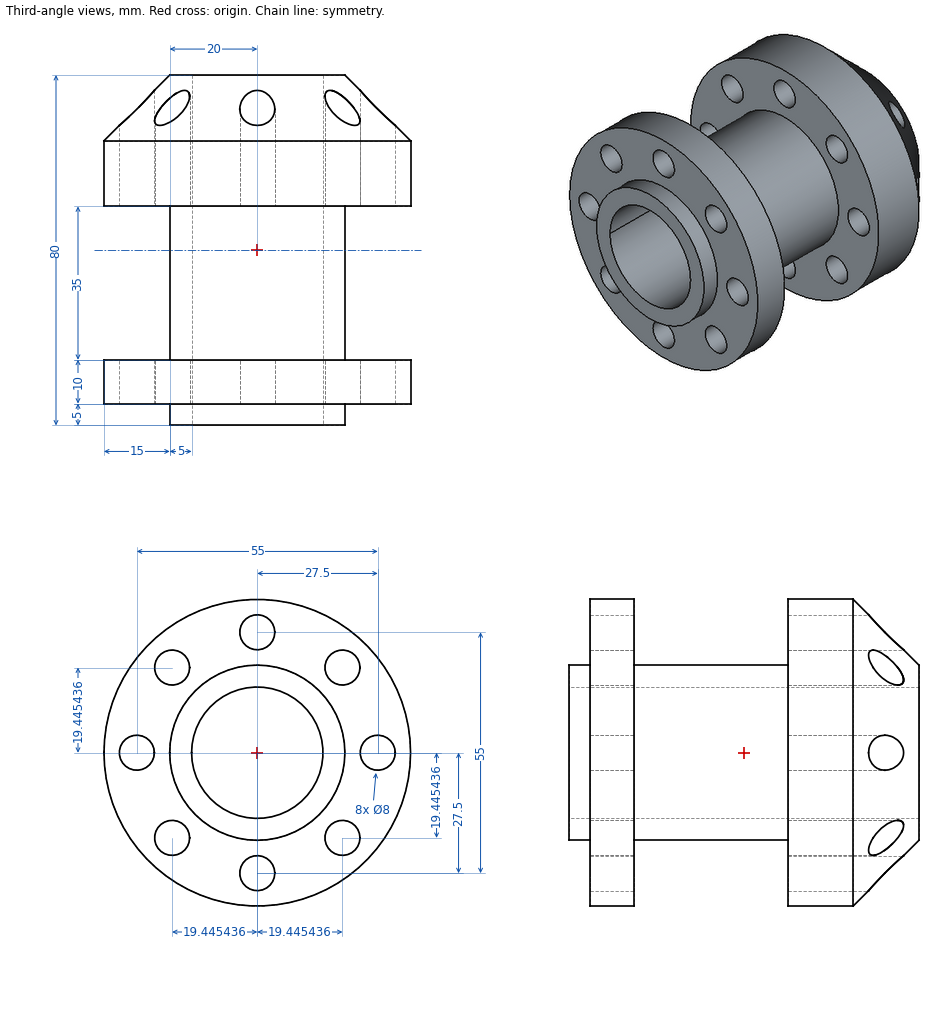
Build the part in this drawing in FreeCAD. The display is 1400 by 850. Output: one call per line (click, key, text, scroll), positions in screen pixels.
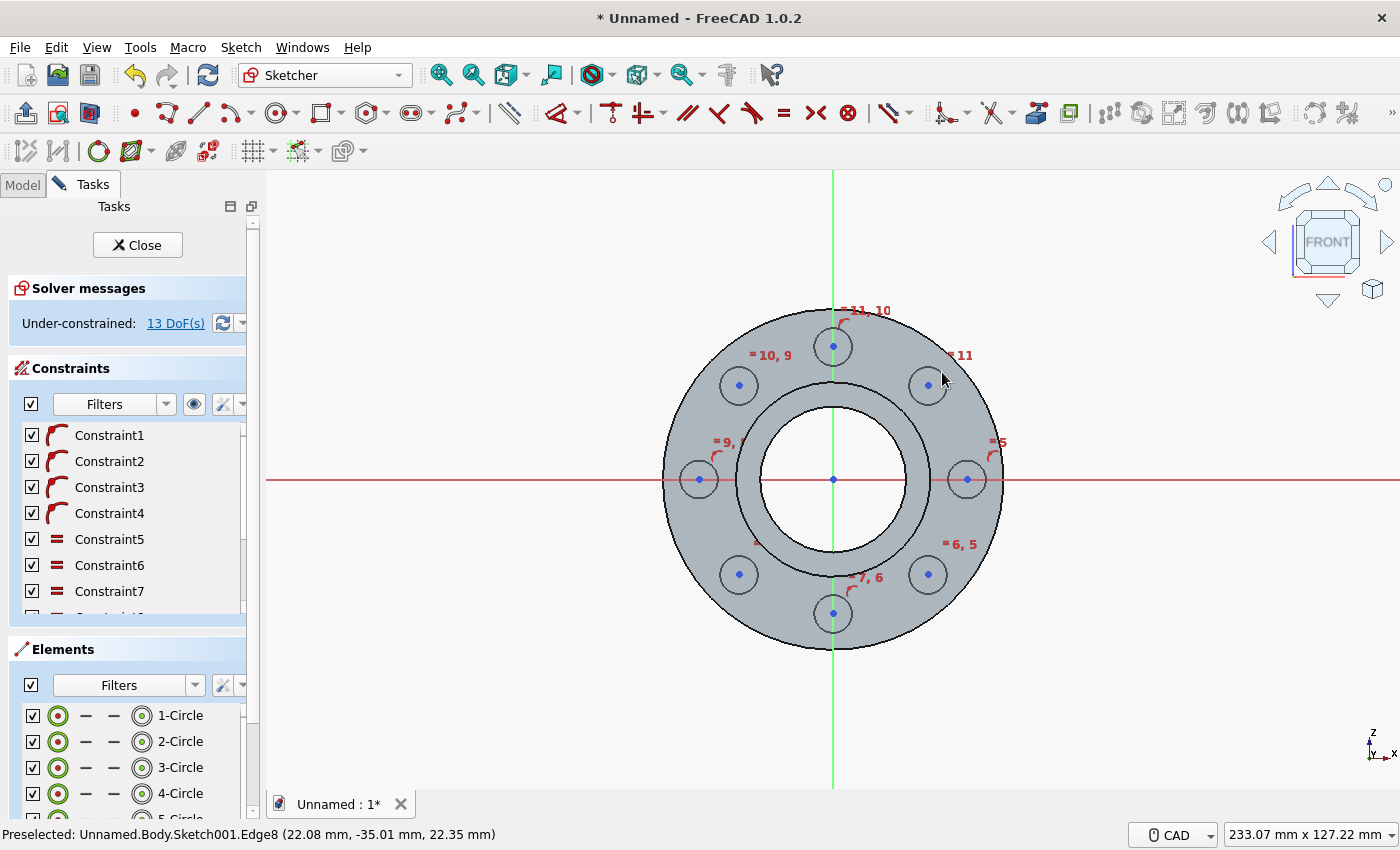
click(928, 575)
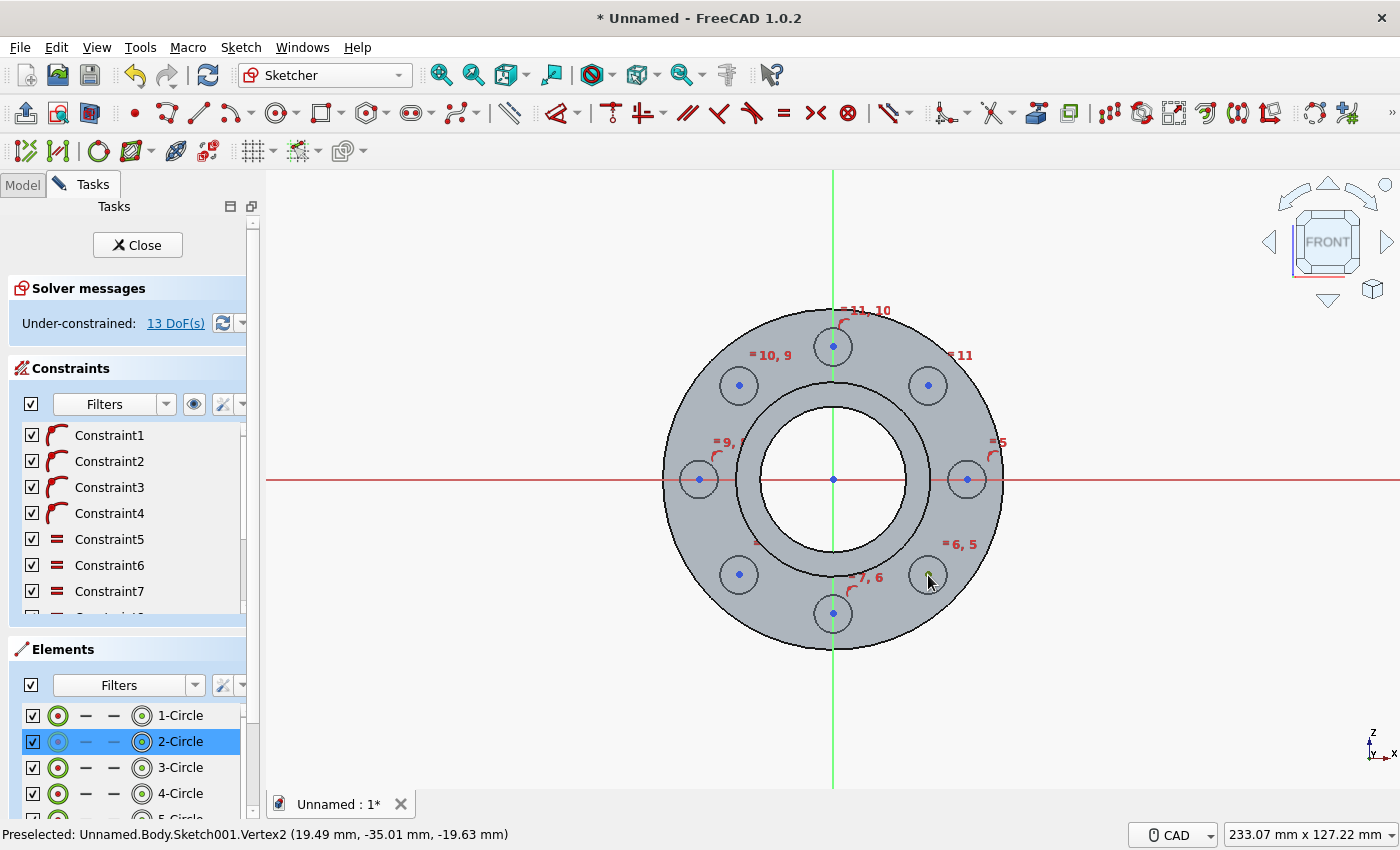
click(739, 575)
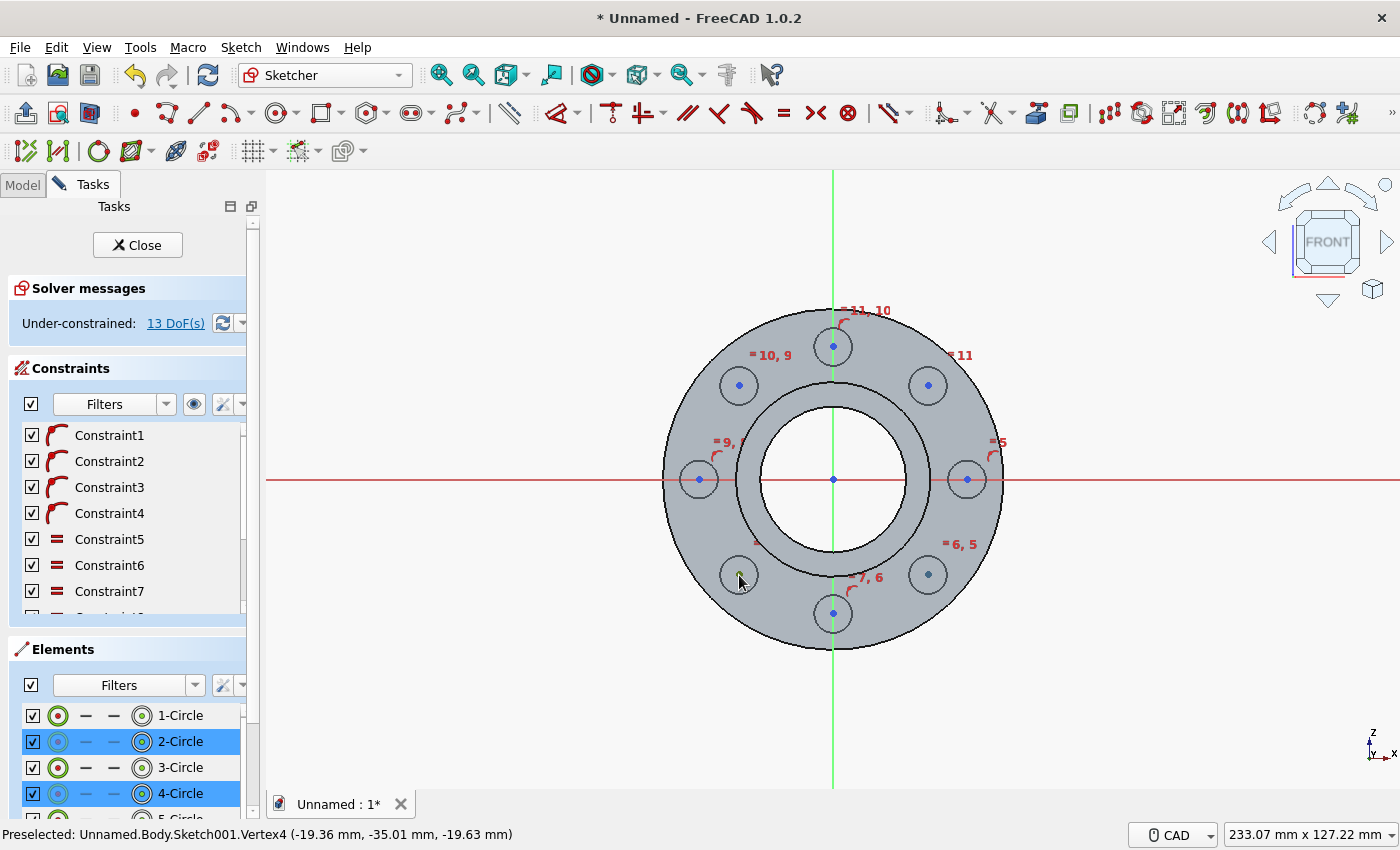
key(h)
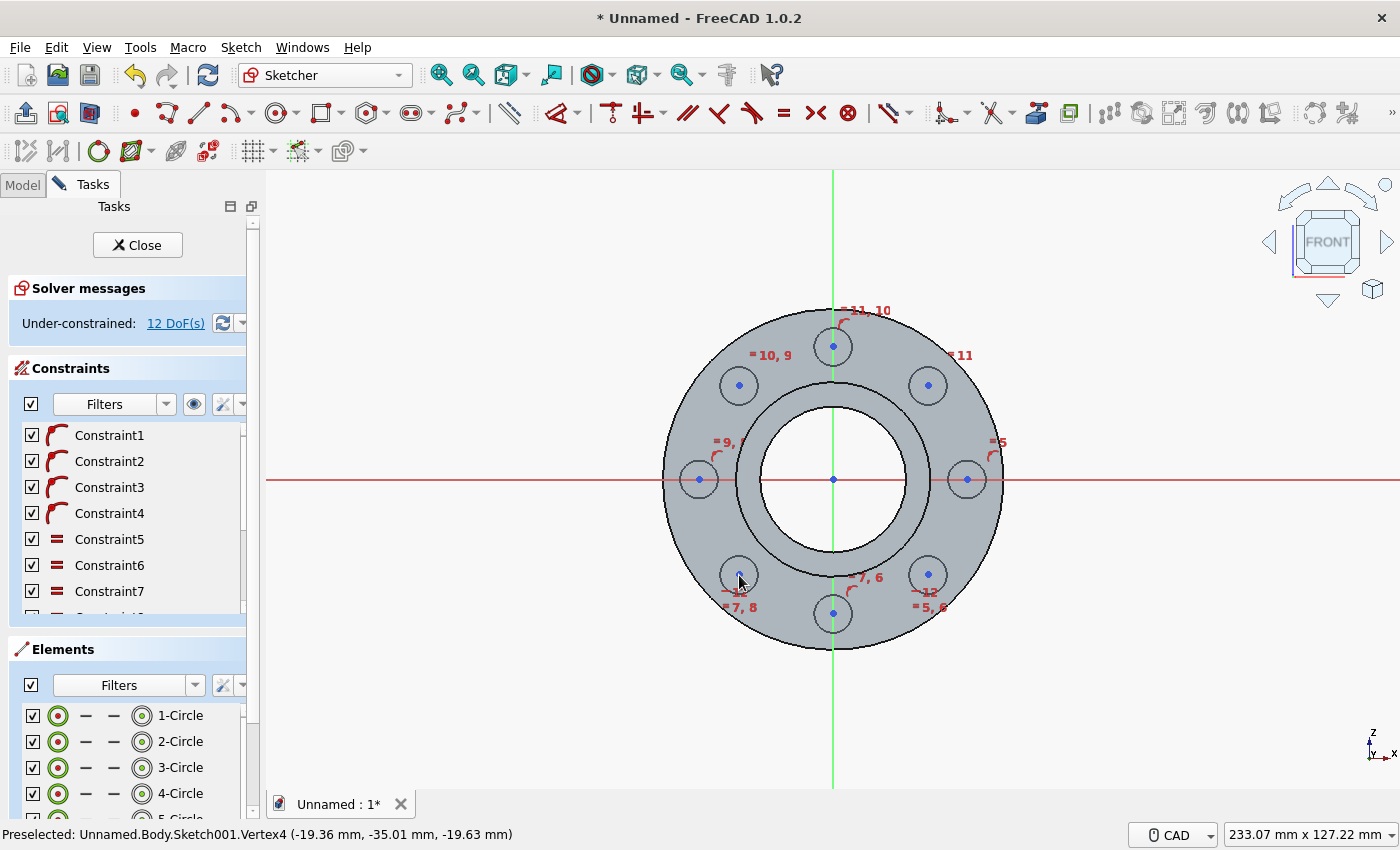
click(739, 575)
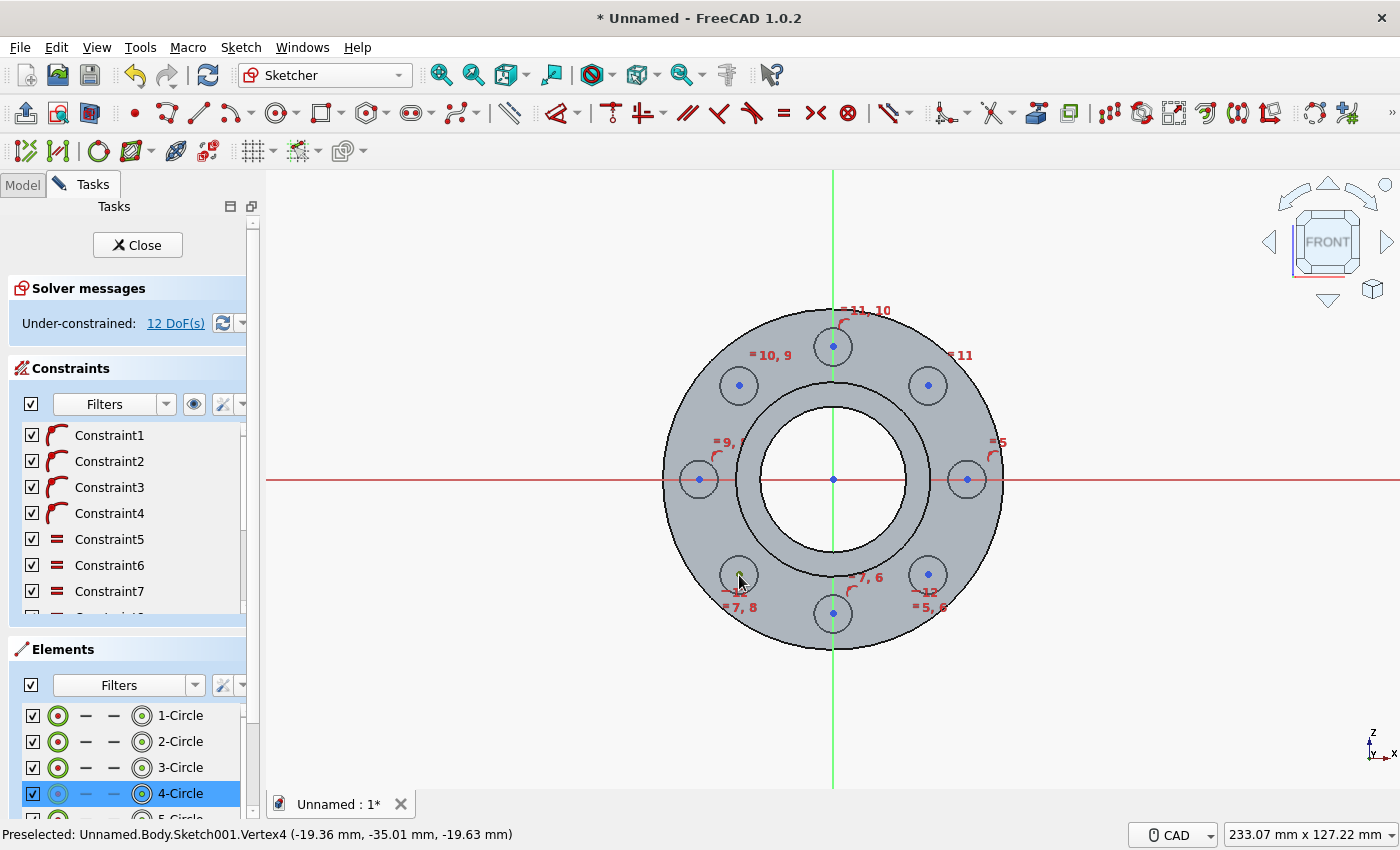
click(739, 386)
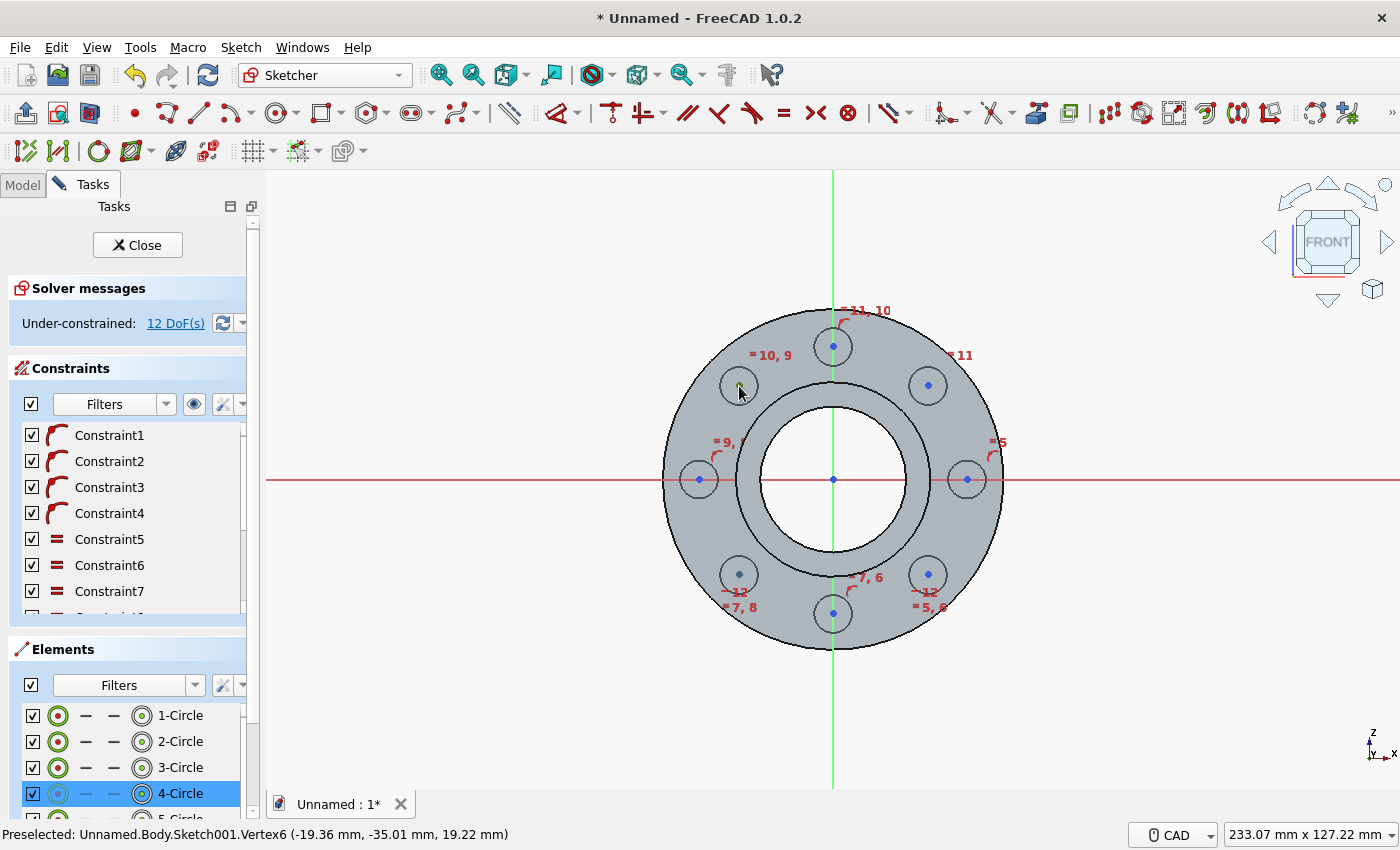
key(v)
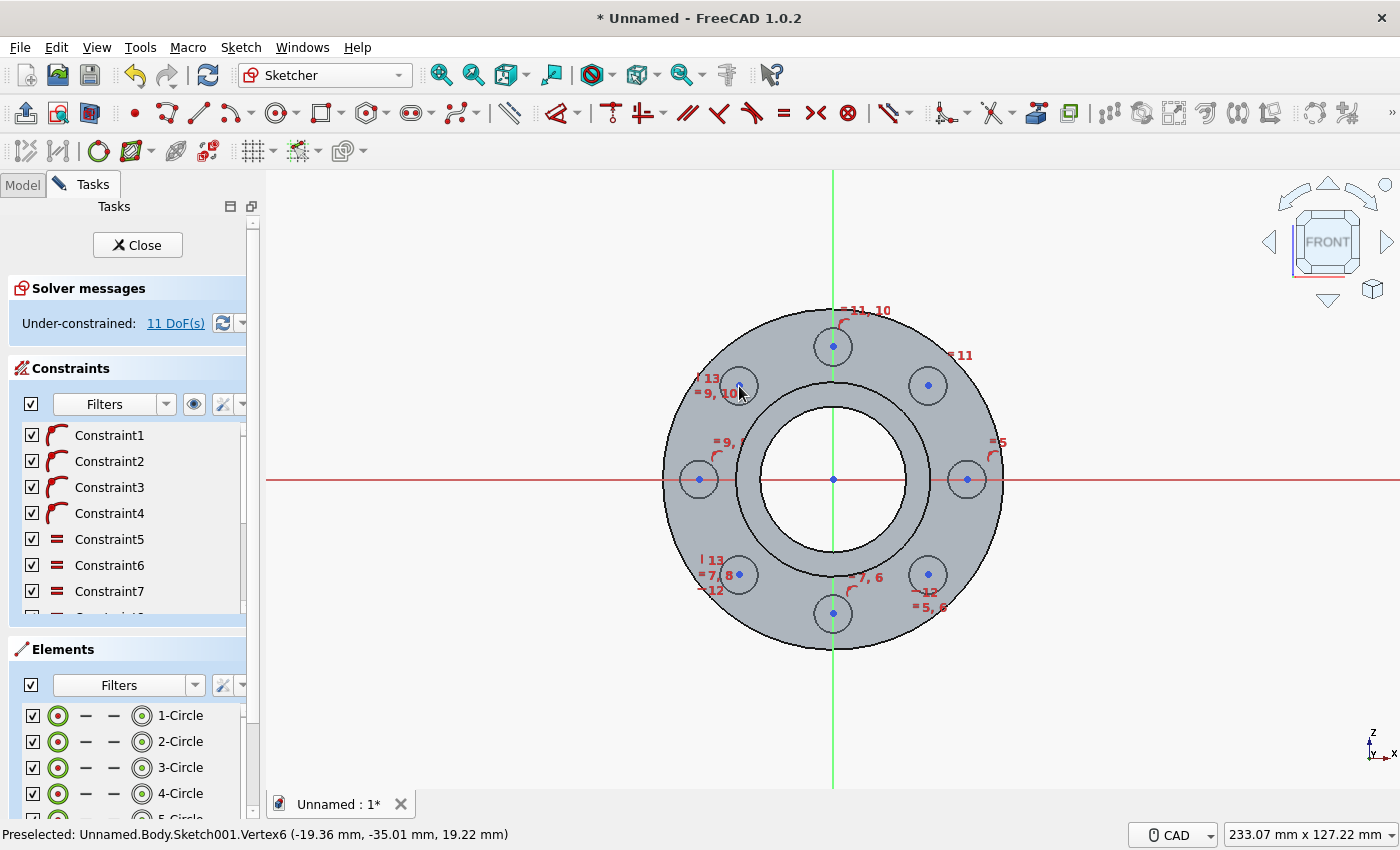
click(928, 575)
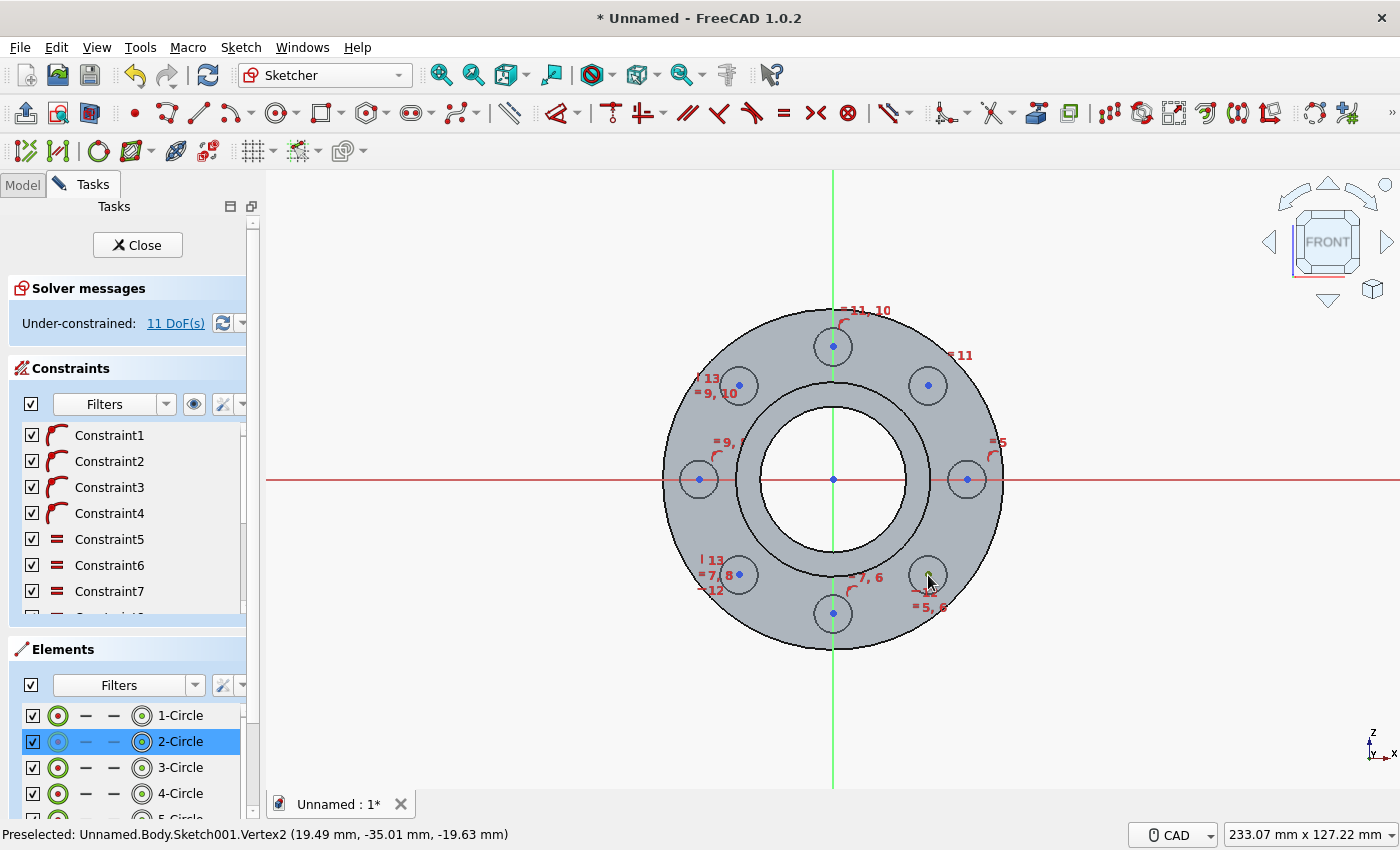
click(928, 386)